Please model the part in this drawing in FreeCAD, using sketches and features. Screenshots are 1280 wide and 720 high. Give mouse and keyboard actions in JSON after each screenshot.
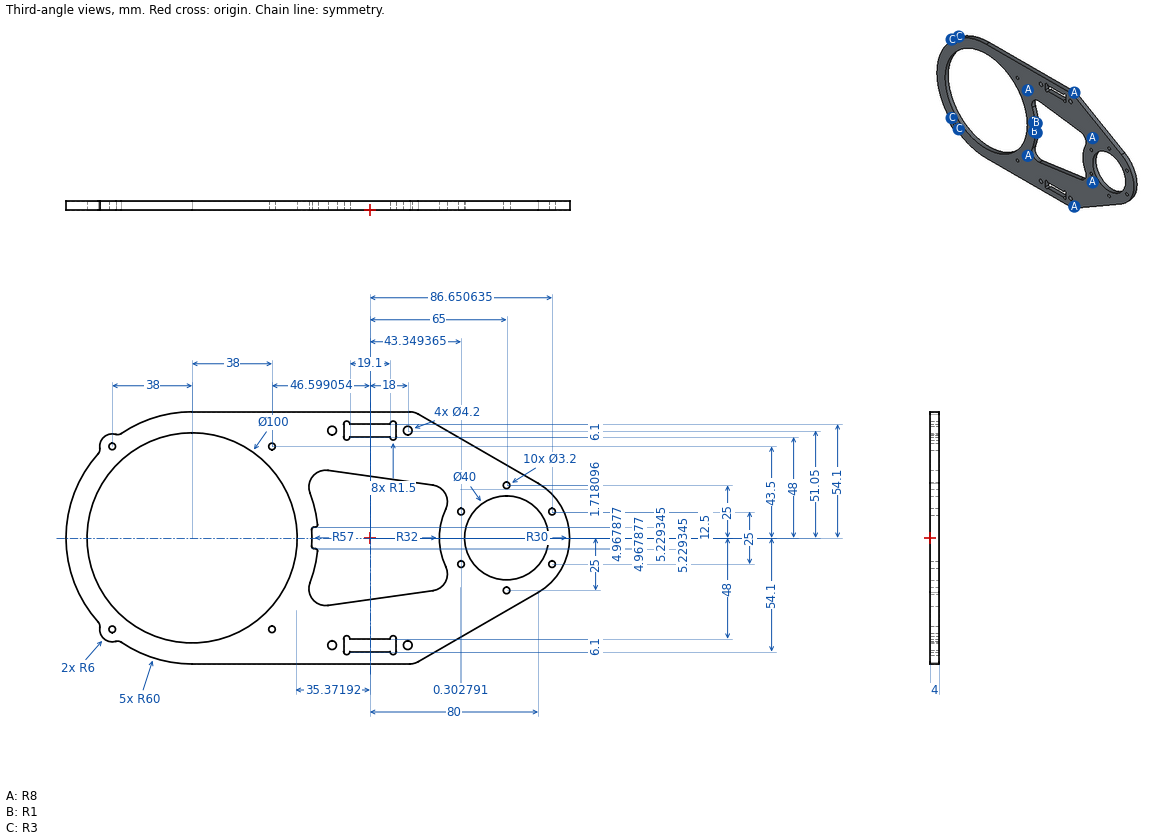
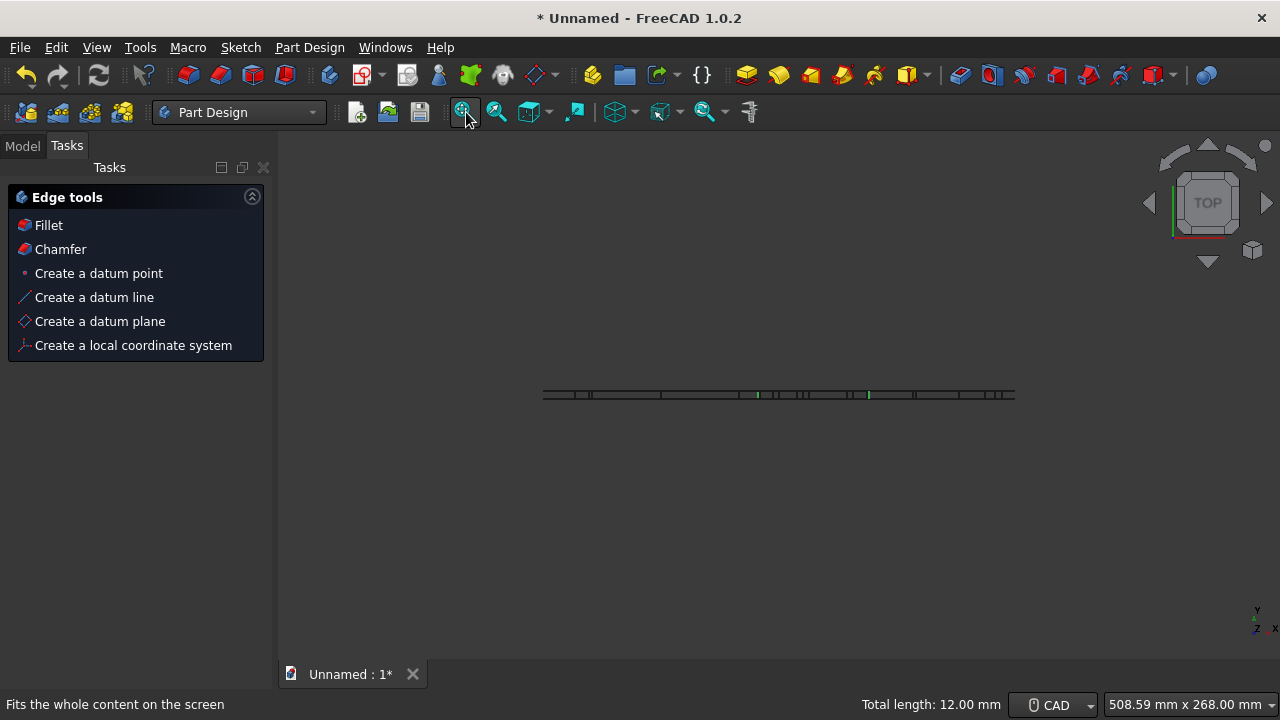
{"action": "key", "text": "1"}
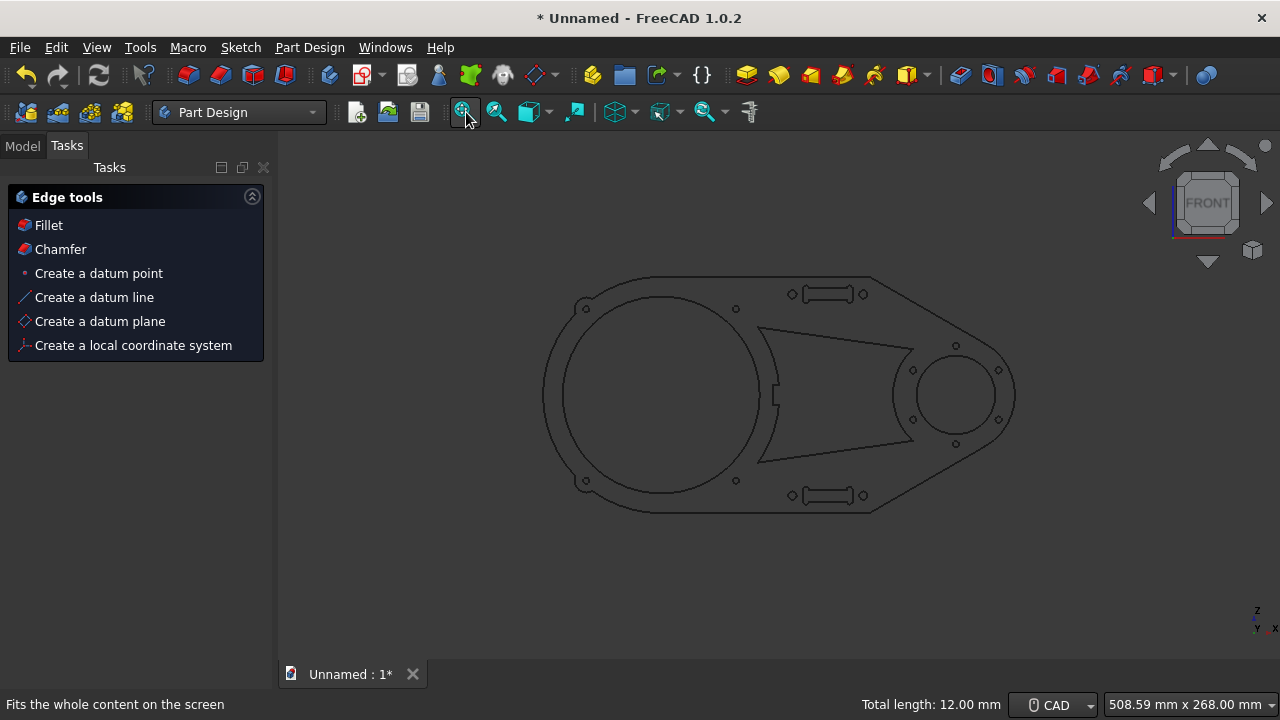
{"action": "scroll", "coordinate": [913, 348], "scroll_direction": "up", "scroll_amount": 9}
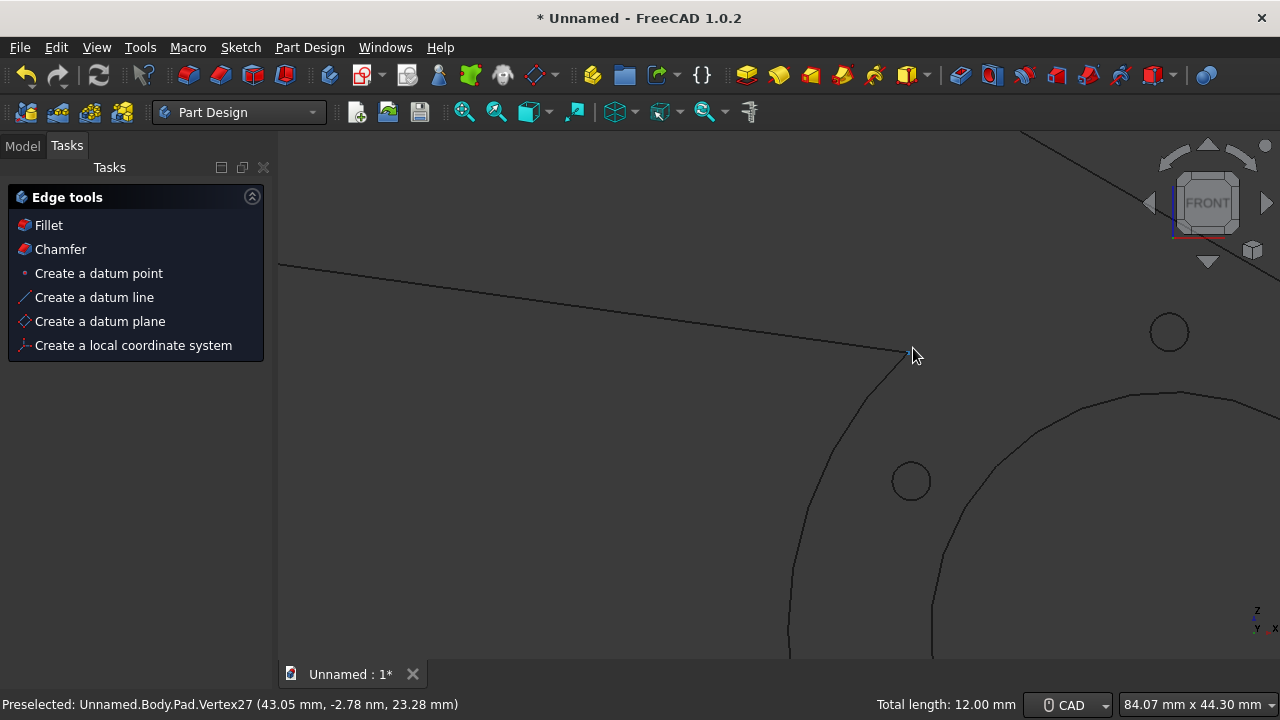
{"action": "left_click", "coordinate": [466, 112]}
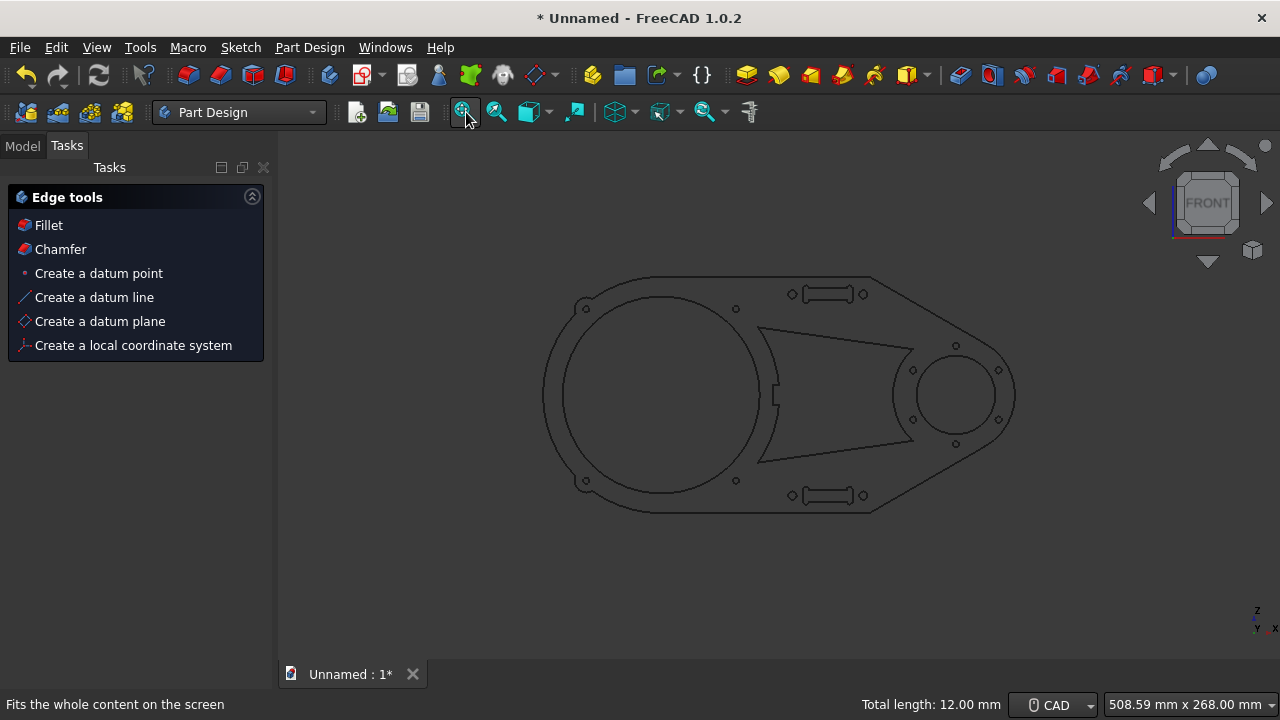
{"action": "key", "text": "3"}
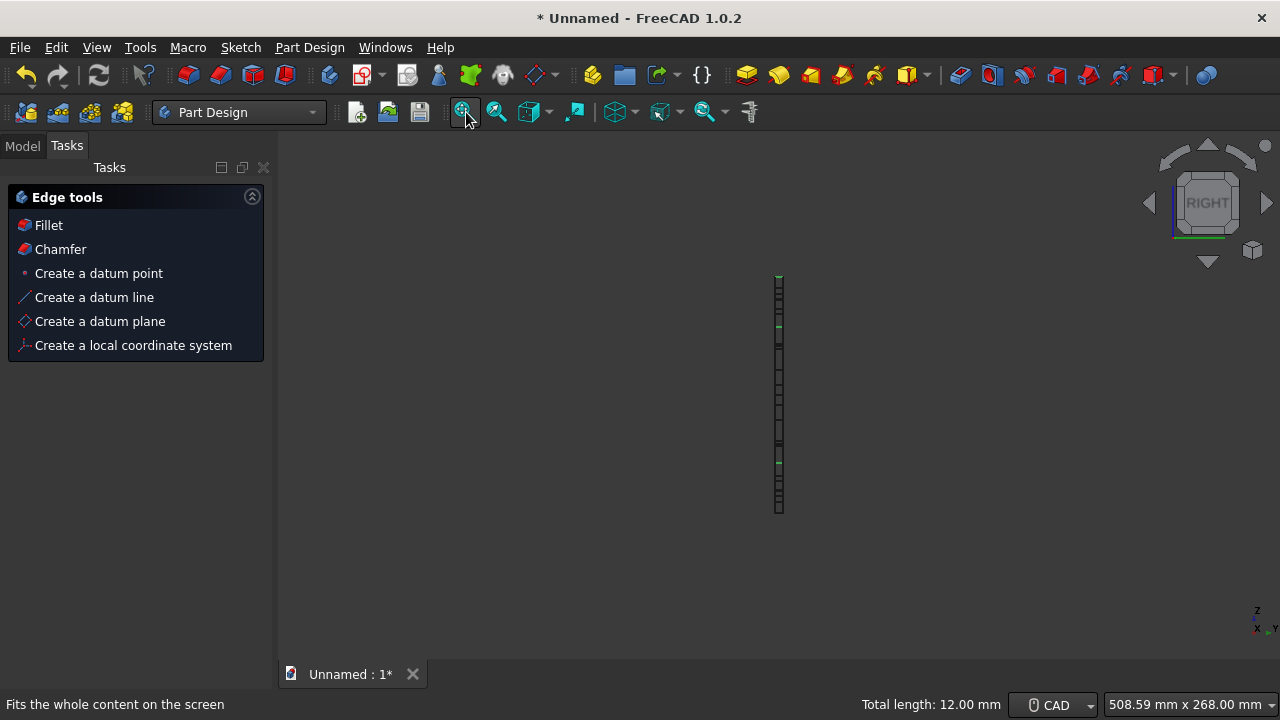
{"action": "left_click", "coordinate": [466, 112]}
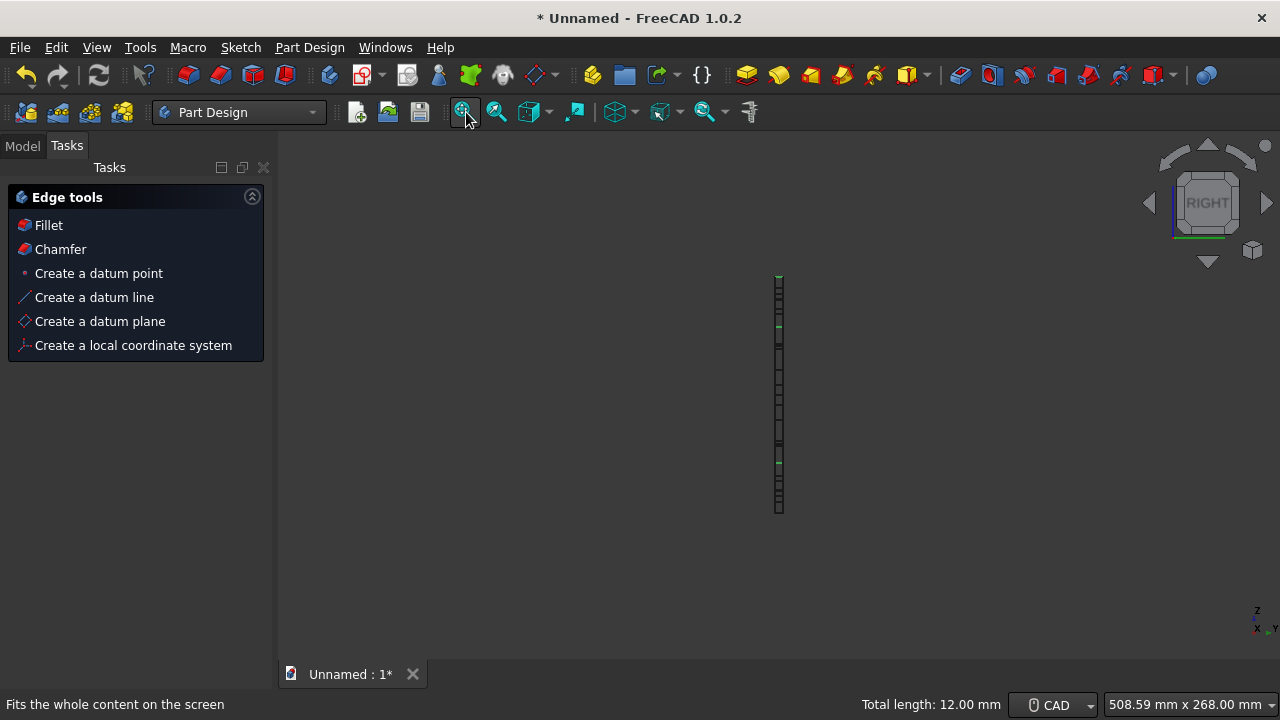
{"action": "scroll", "coordinate": [779, 348], "scroll_direction": "up", "scroll_amount": 9}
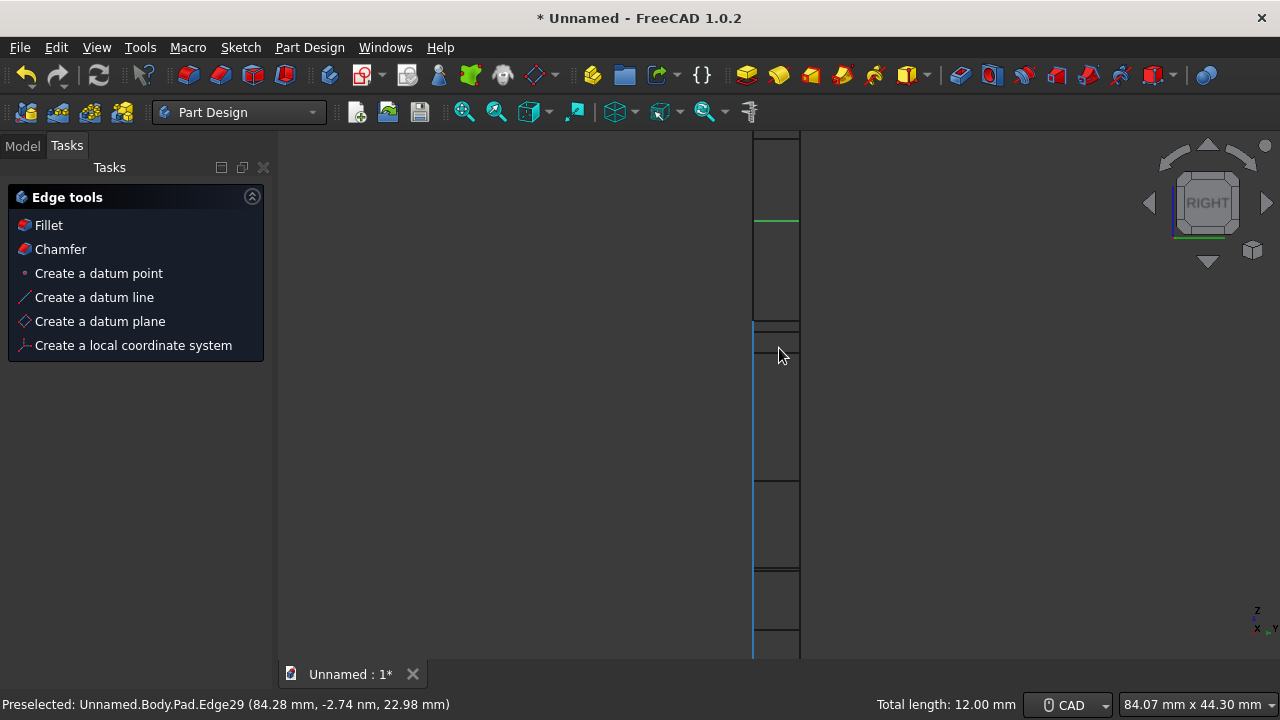
{"action": "left_click", "coordinate": [776, 352], "text": "ctrl"}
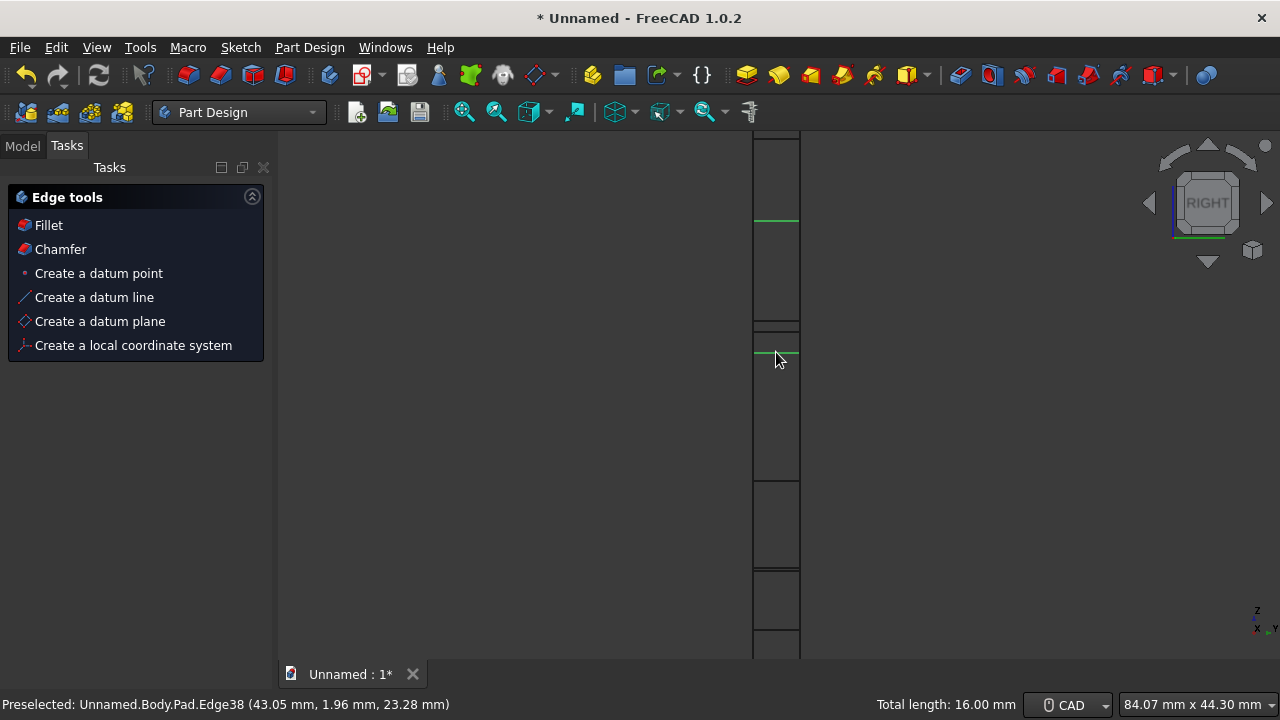
{"action": "left_click", "coordinate": [466, 112]}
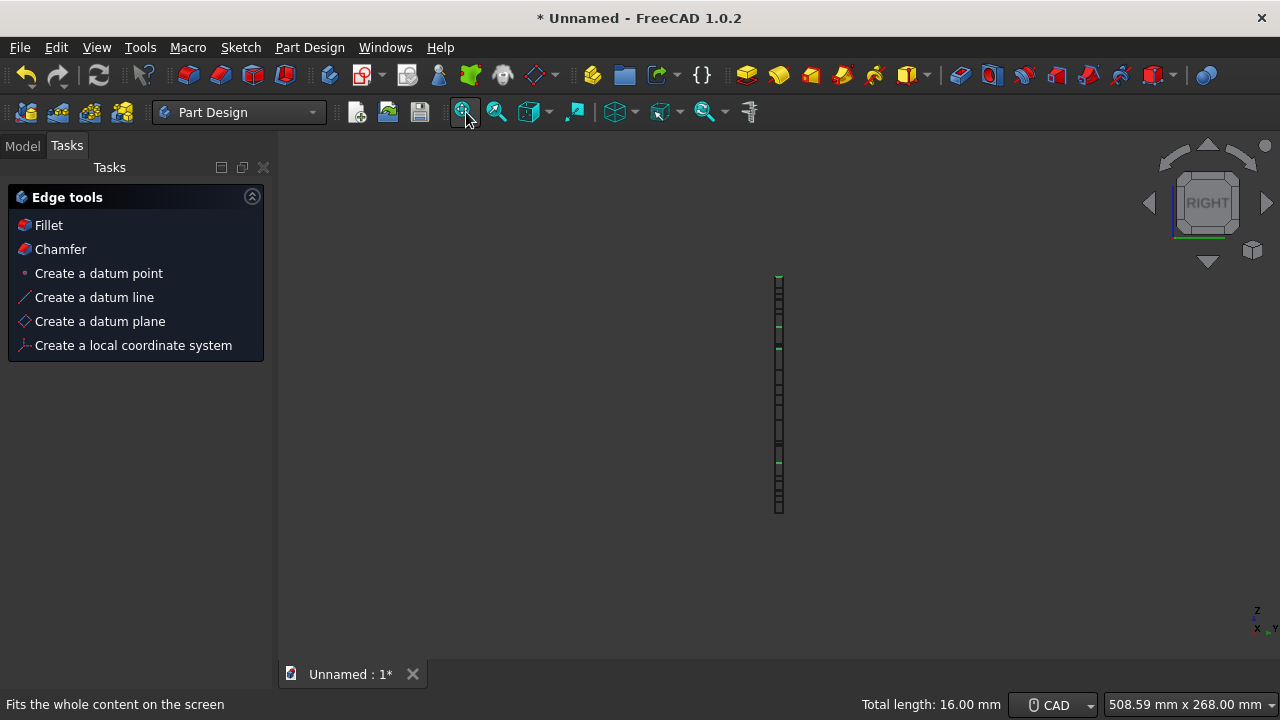
{"action": "key", "text": "5"}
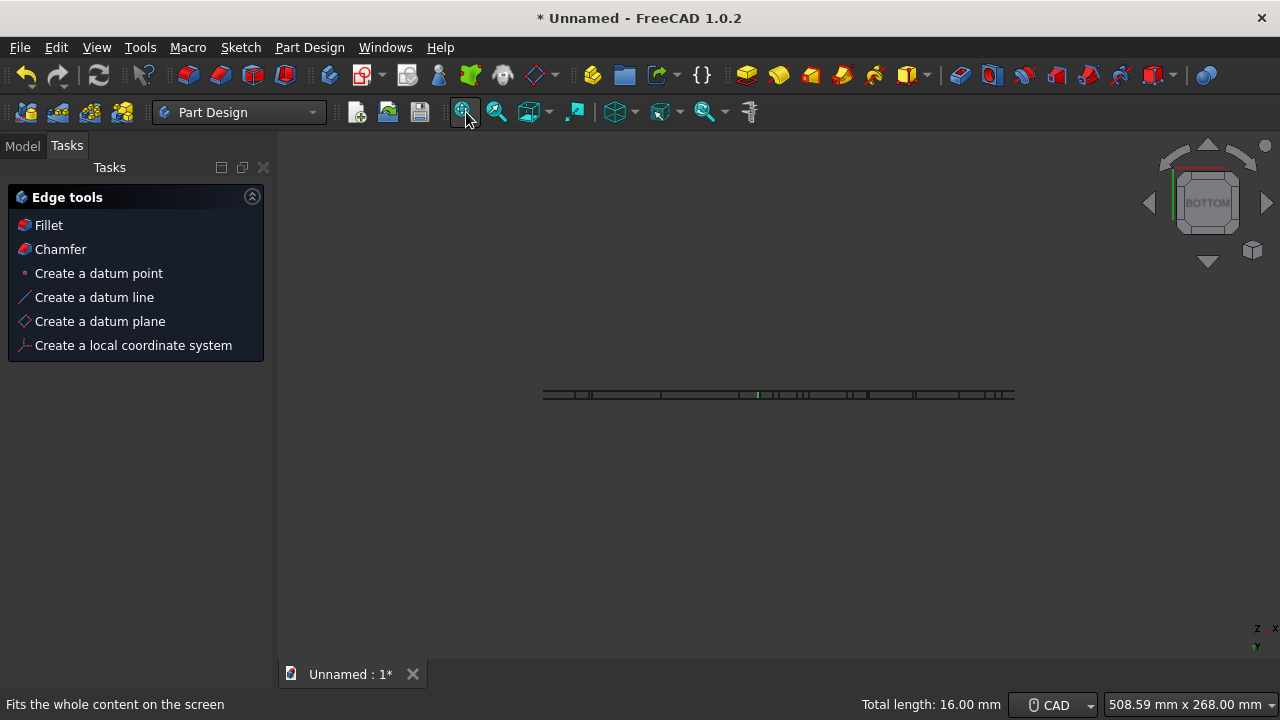
{"action": "left_click", "coordinate": [869, 397], "text": "ctrl"}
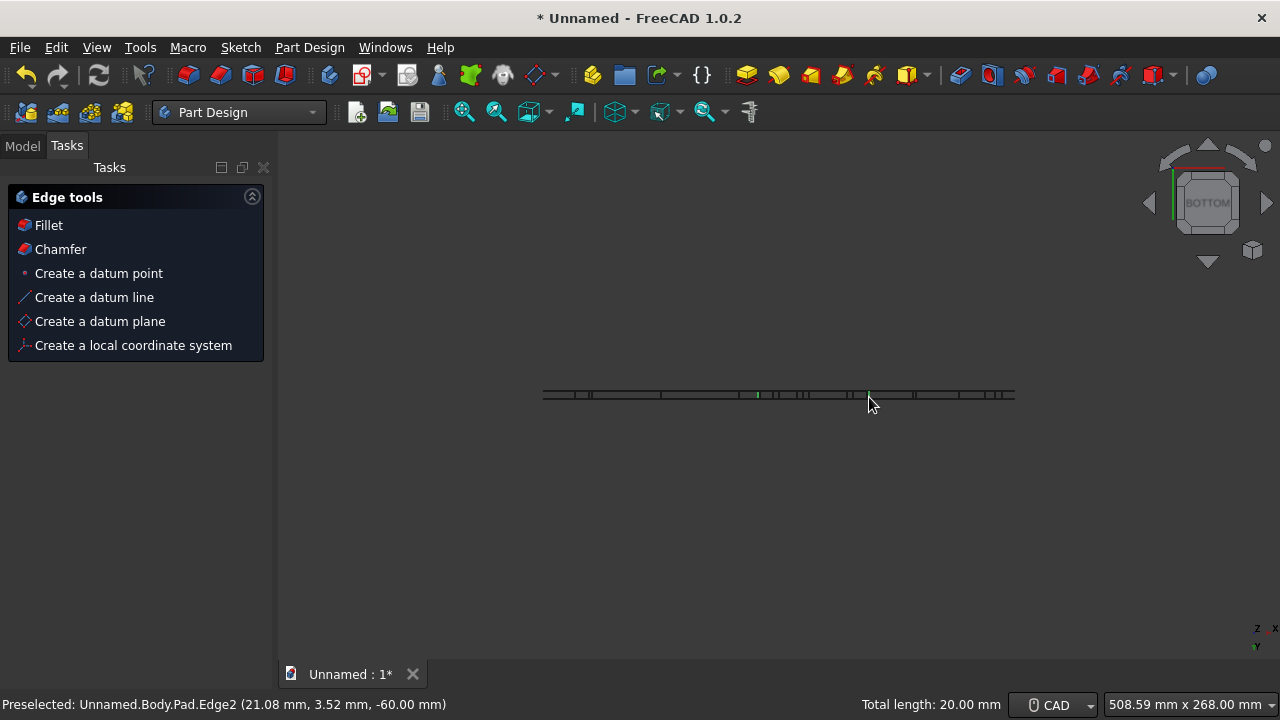
{"action": "scroll", "coordinate": [913, 394], "scroll_direction": "up", "scroll_amount": 9}